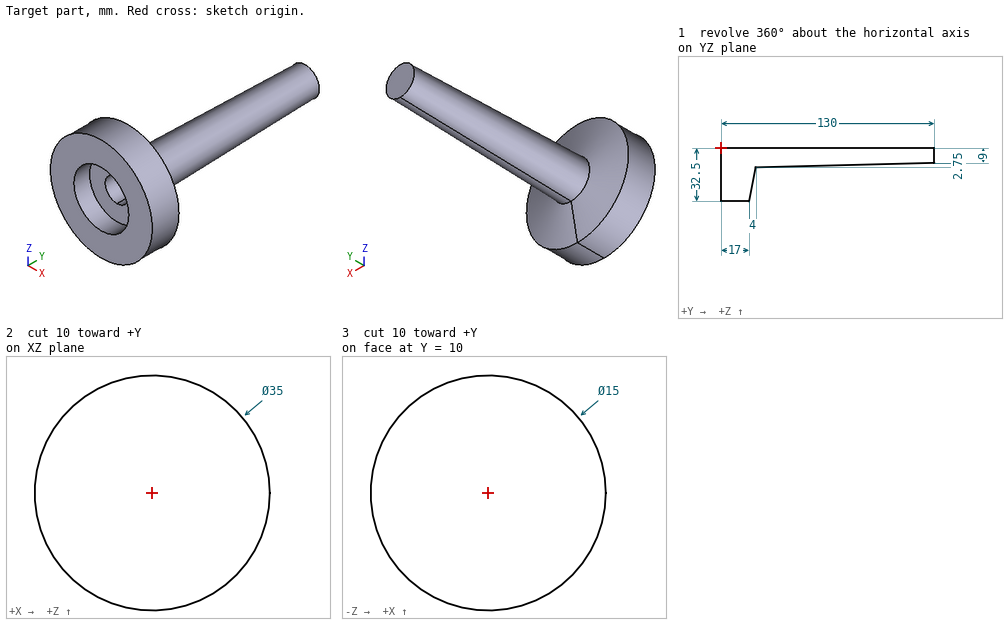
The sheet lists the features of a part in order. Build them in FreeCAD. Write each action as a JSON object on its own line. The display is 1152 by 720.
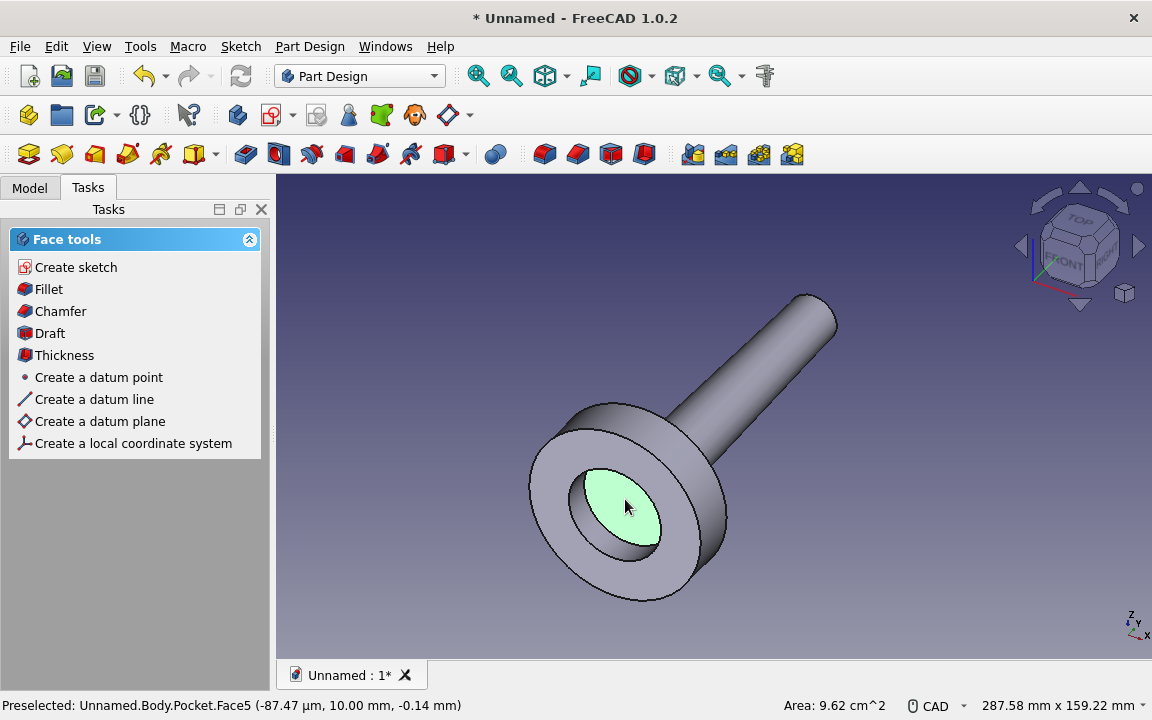
{"action": "left_click", "coordinate": [270, 116]}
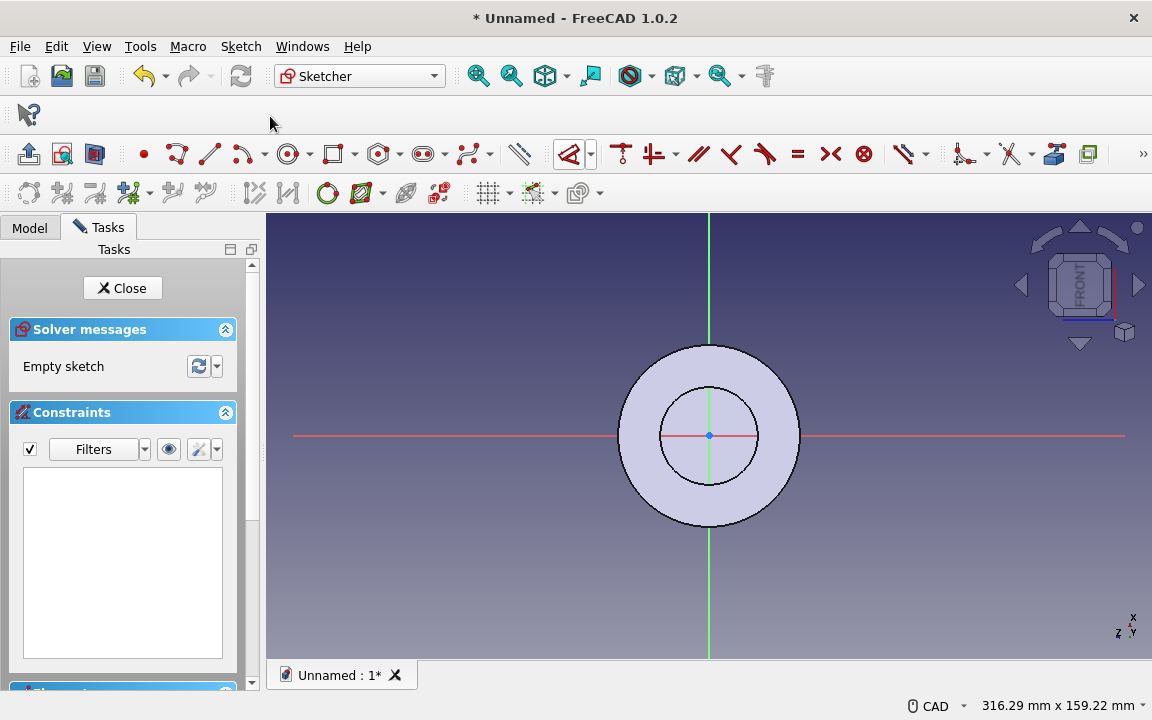
{"action": "left_click", "coordinate": [95, 154]}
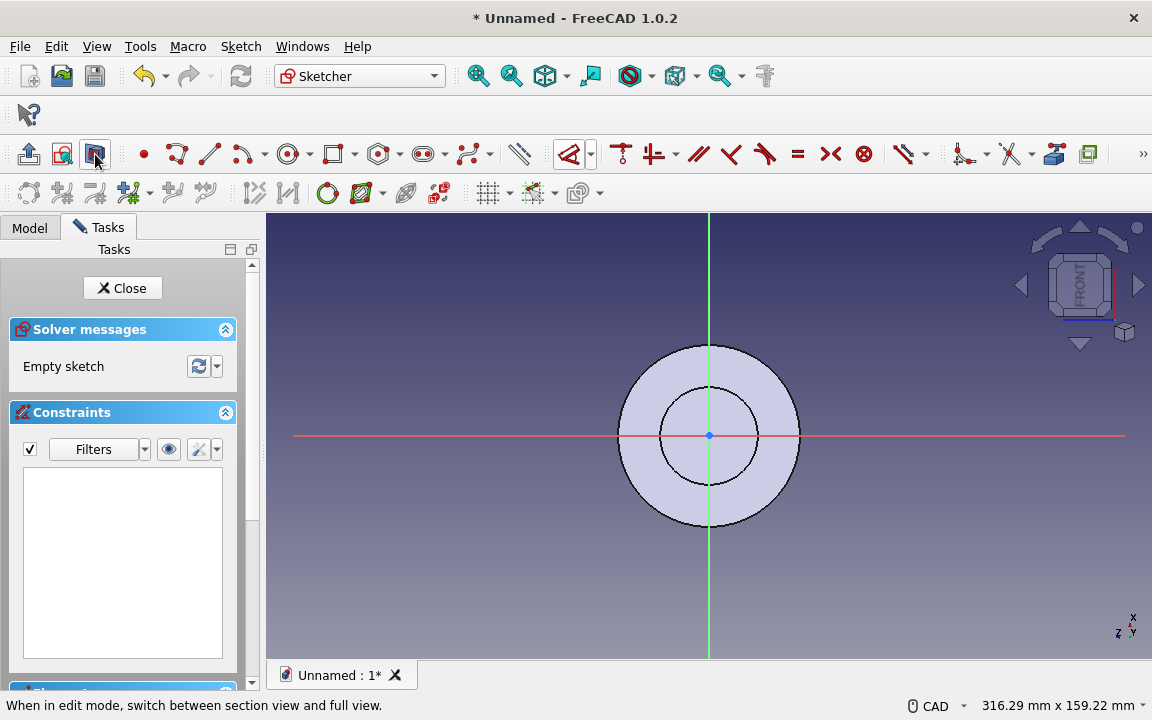
{"action": "scroll", "coordinate": [723, 436], "scroll_direction": "up", "scroll_amount": 9}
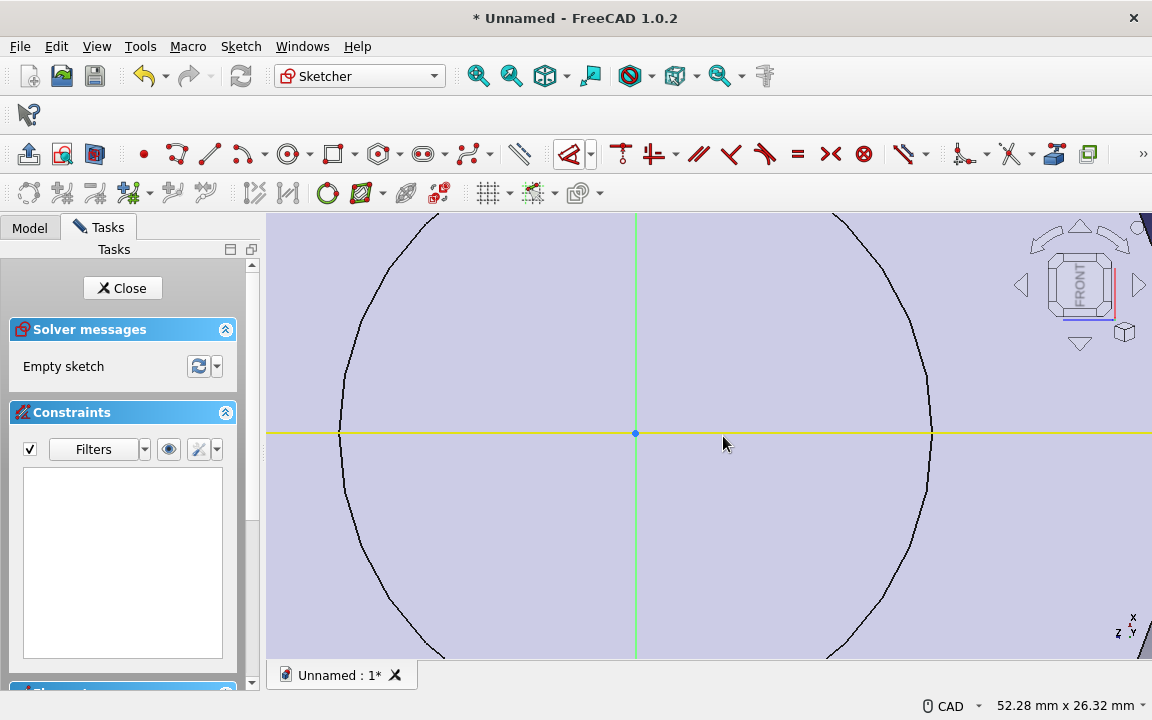
{"action": "left_click", "coordinate": [288, 154]}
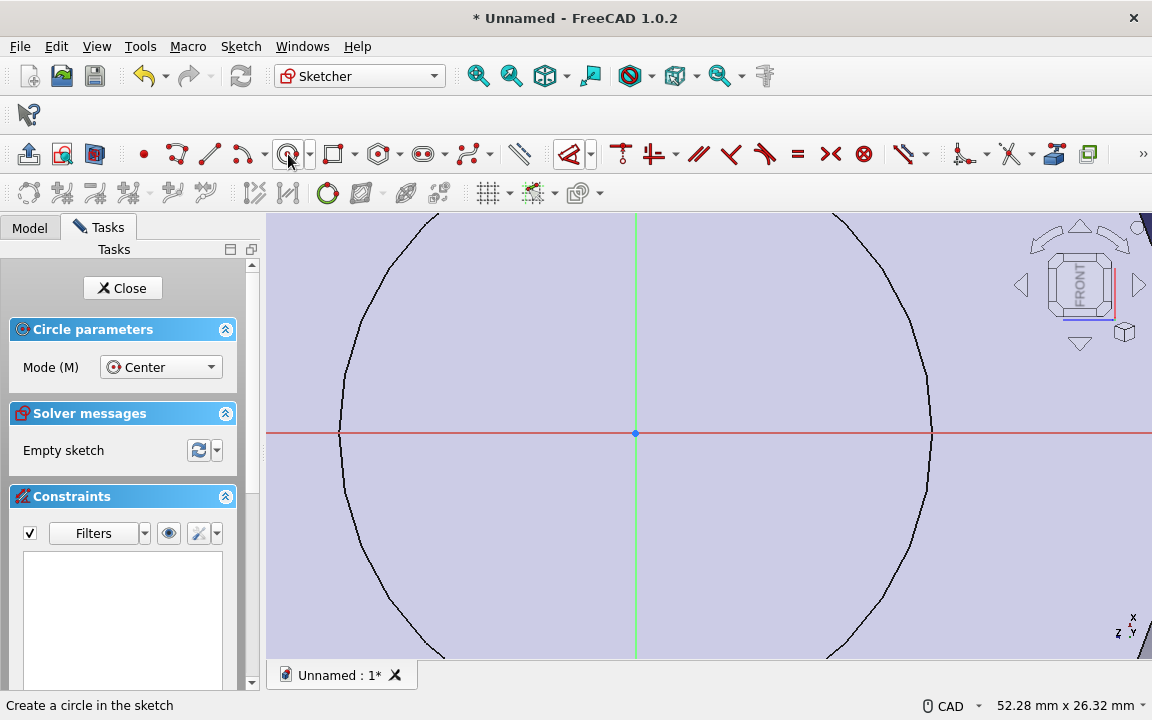
{"action": "left_click", "coordinate": [636, 433]}
{"action": "mouse_move", "coordinate": [726, 344]}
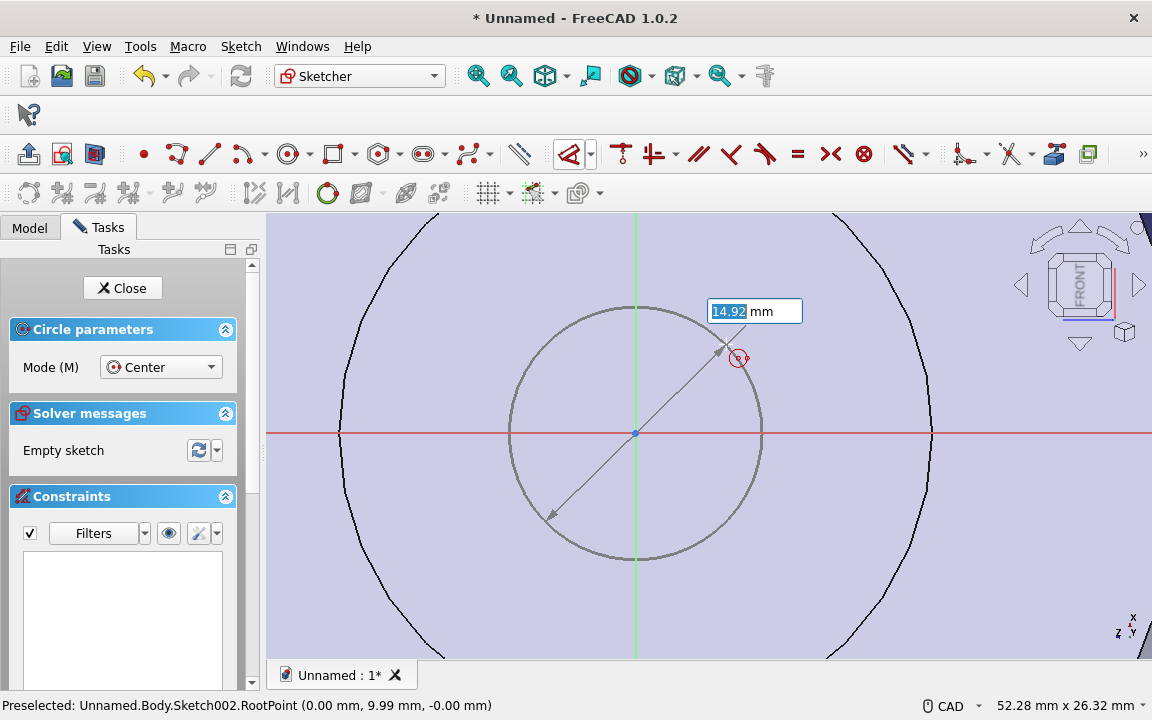
{"action": "type", "text": "15"}
{"action": "key", "text": "Return"}
{"action": "key", "text": "Escape"}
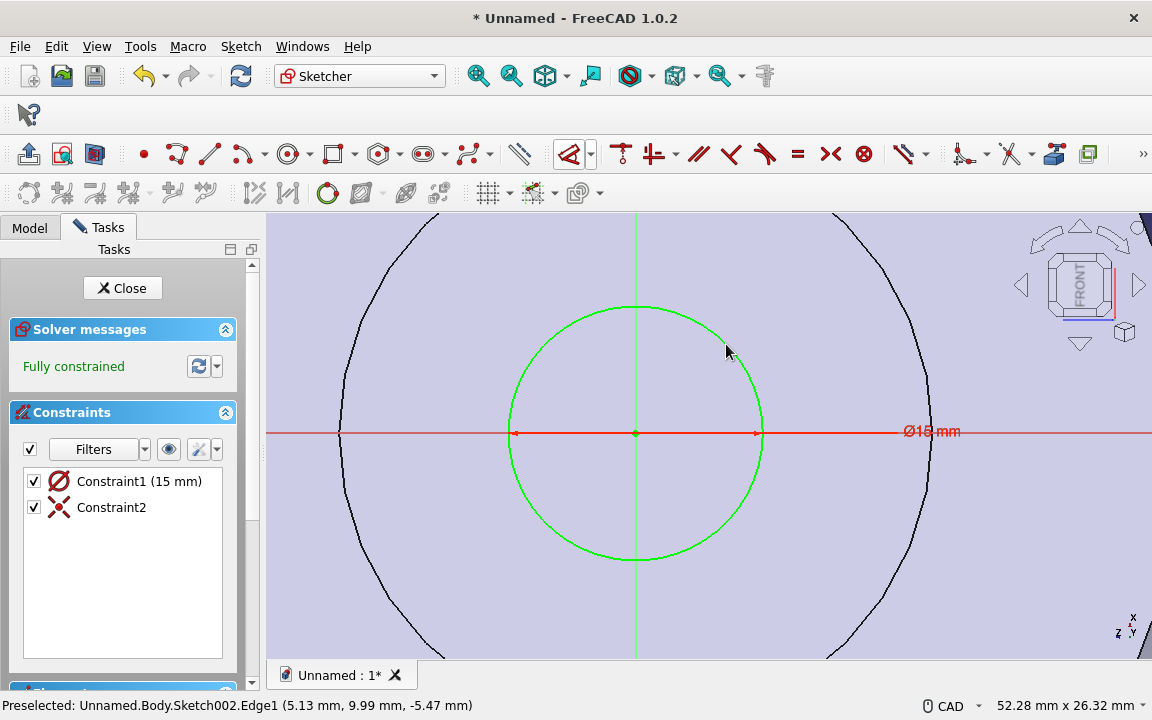
{"action": "left_click", "coordinate": [123, 288]}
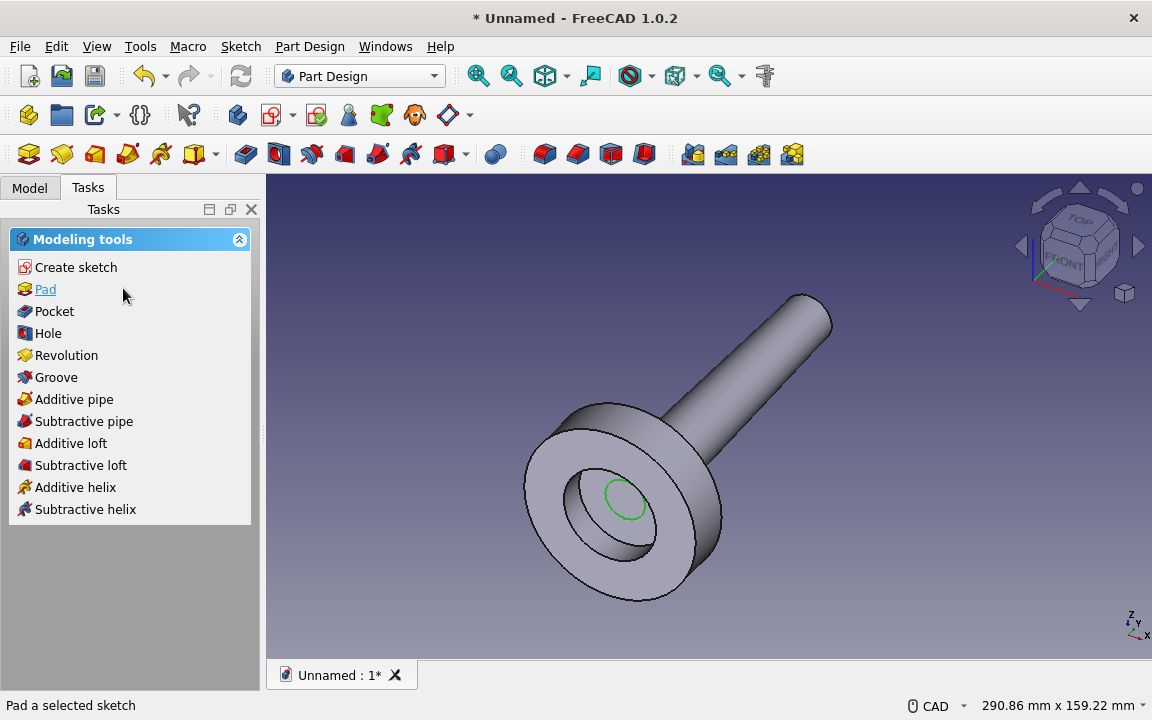
{"action": "left_click", "coordinate": [246, 154]}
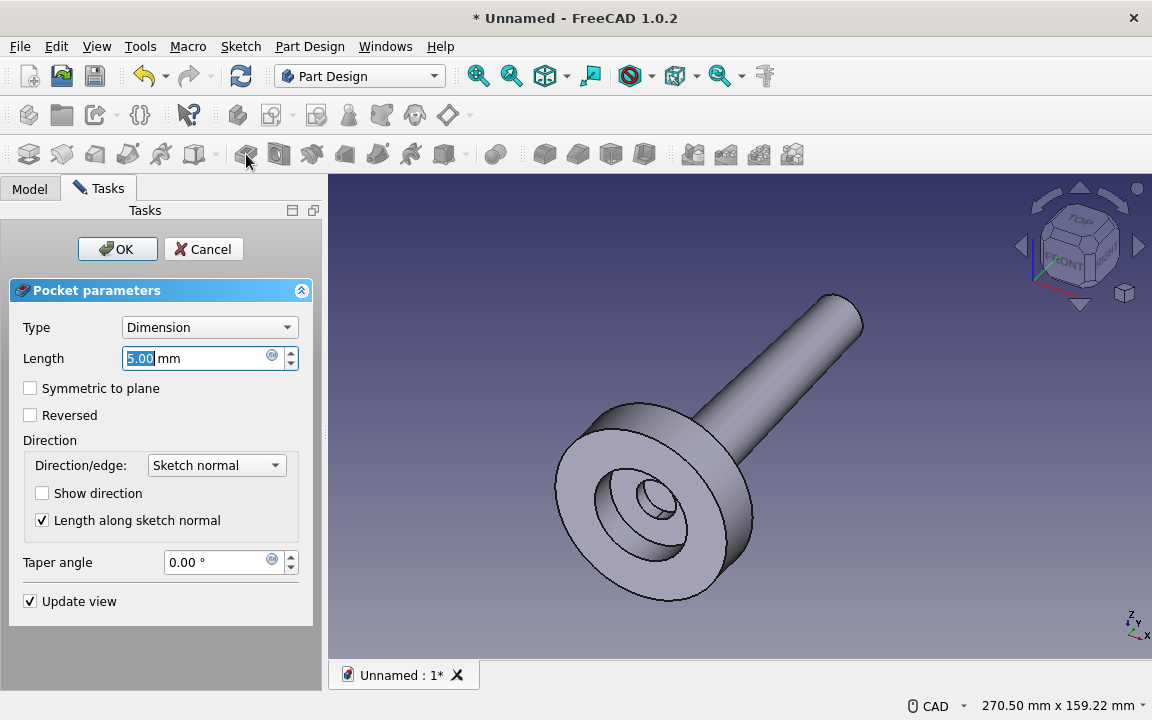
{"action": "type", "text": "10"}
{"action": "key", "text": "Tab"}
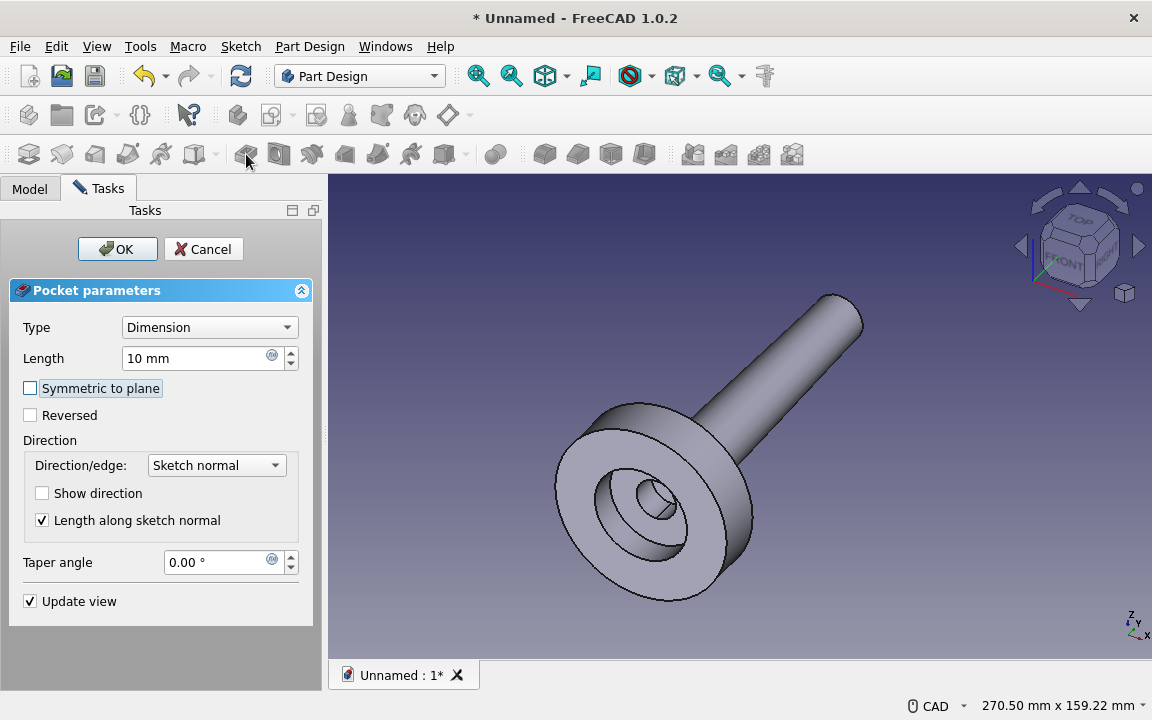
{"action": "left_click", "coordinate": [118, 249]}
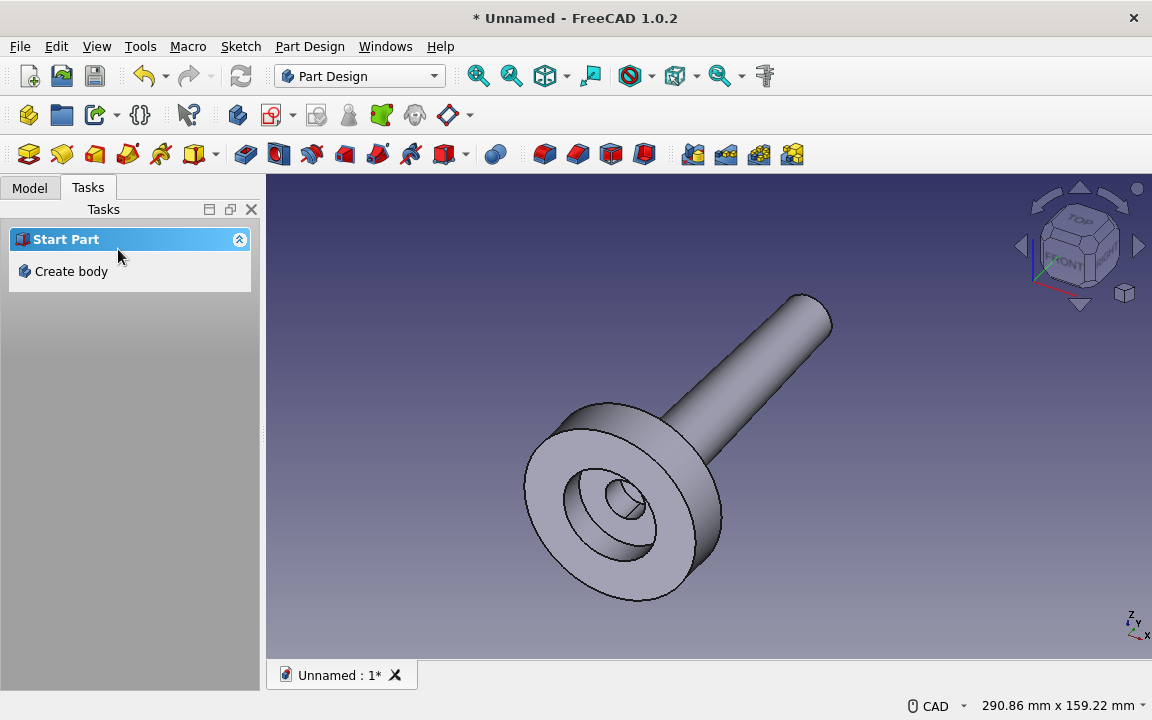
{"action": "key", "text": "0"}